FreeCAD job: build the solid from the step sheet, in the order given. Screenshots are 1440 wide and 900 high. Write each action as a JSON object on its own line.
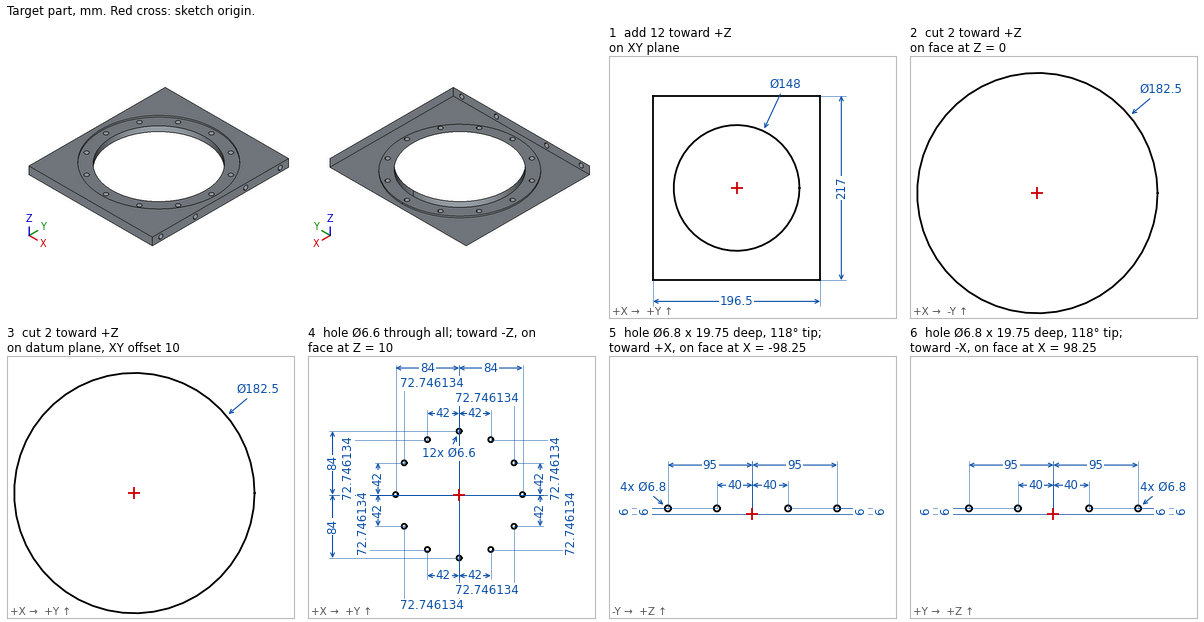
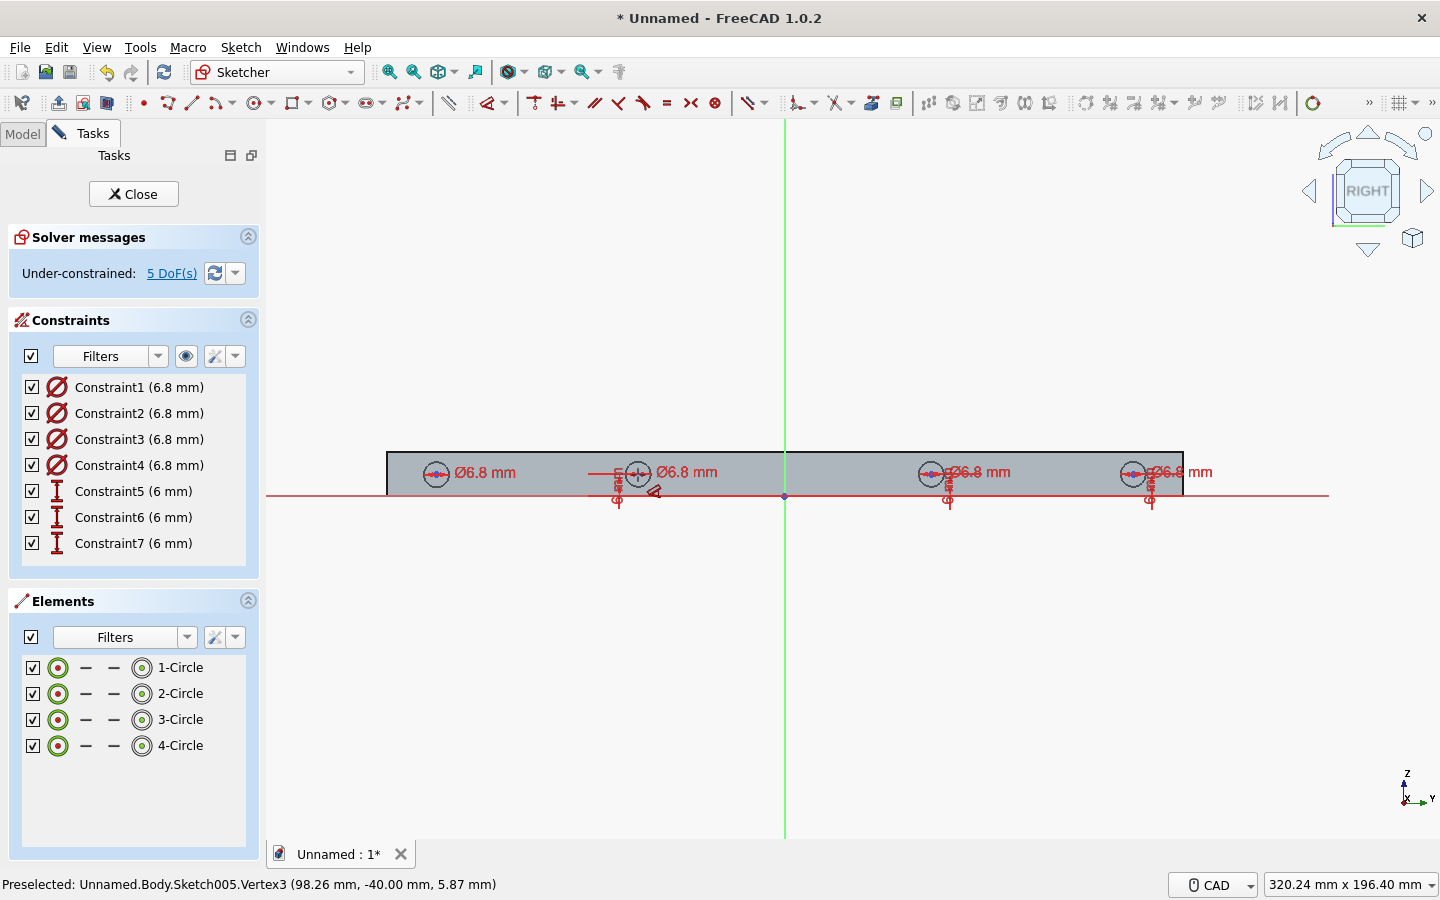
{"action": "scroll", "coordinate": [437, 475], "scroll_direction": "up", "scroll_amount": 3}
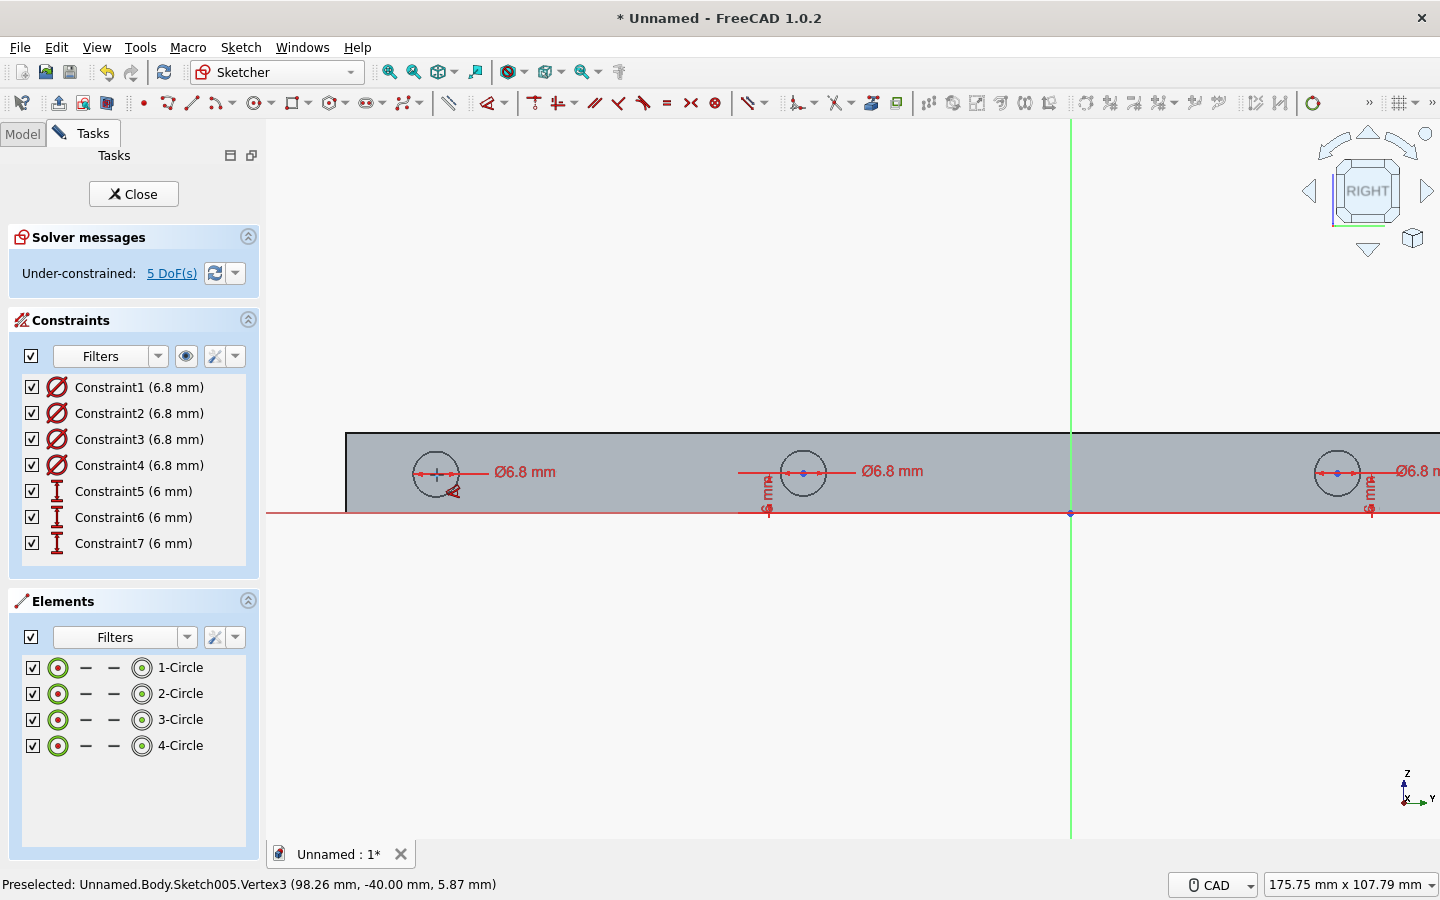
{"action": "left_click", "coordinate": [436, 474]}
{"action": "left_click", "coordinate": [402, 494]}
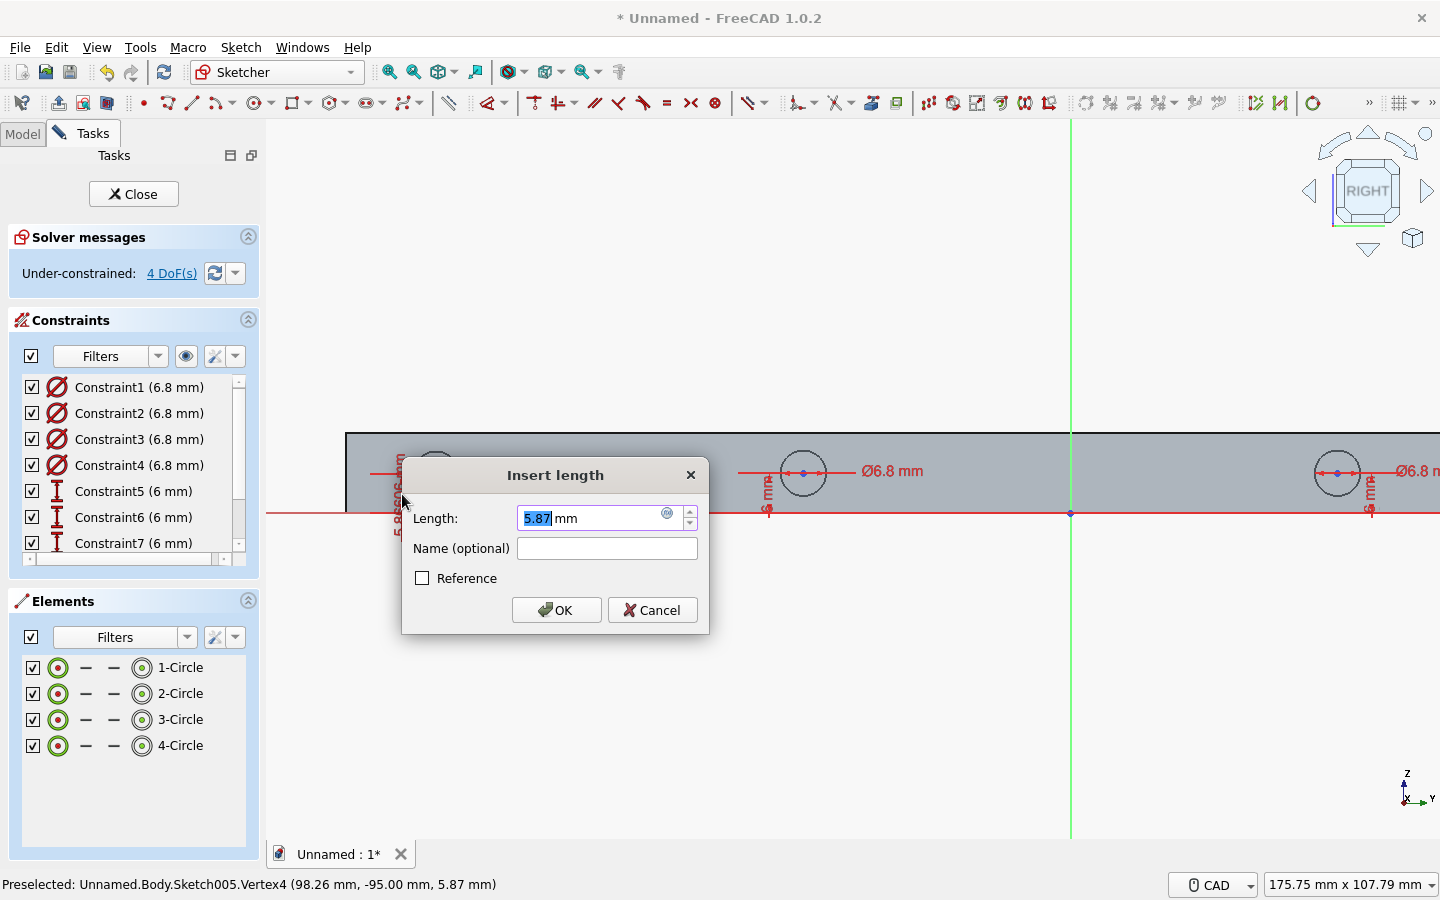
{"action": "type", "text": "6"}
{"action": "key", "text": "Return"}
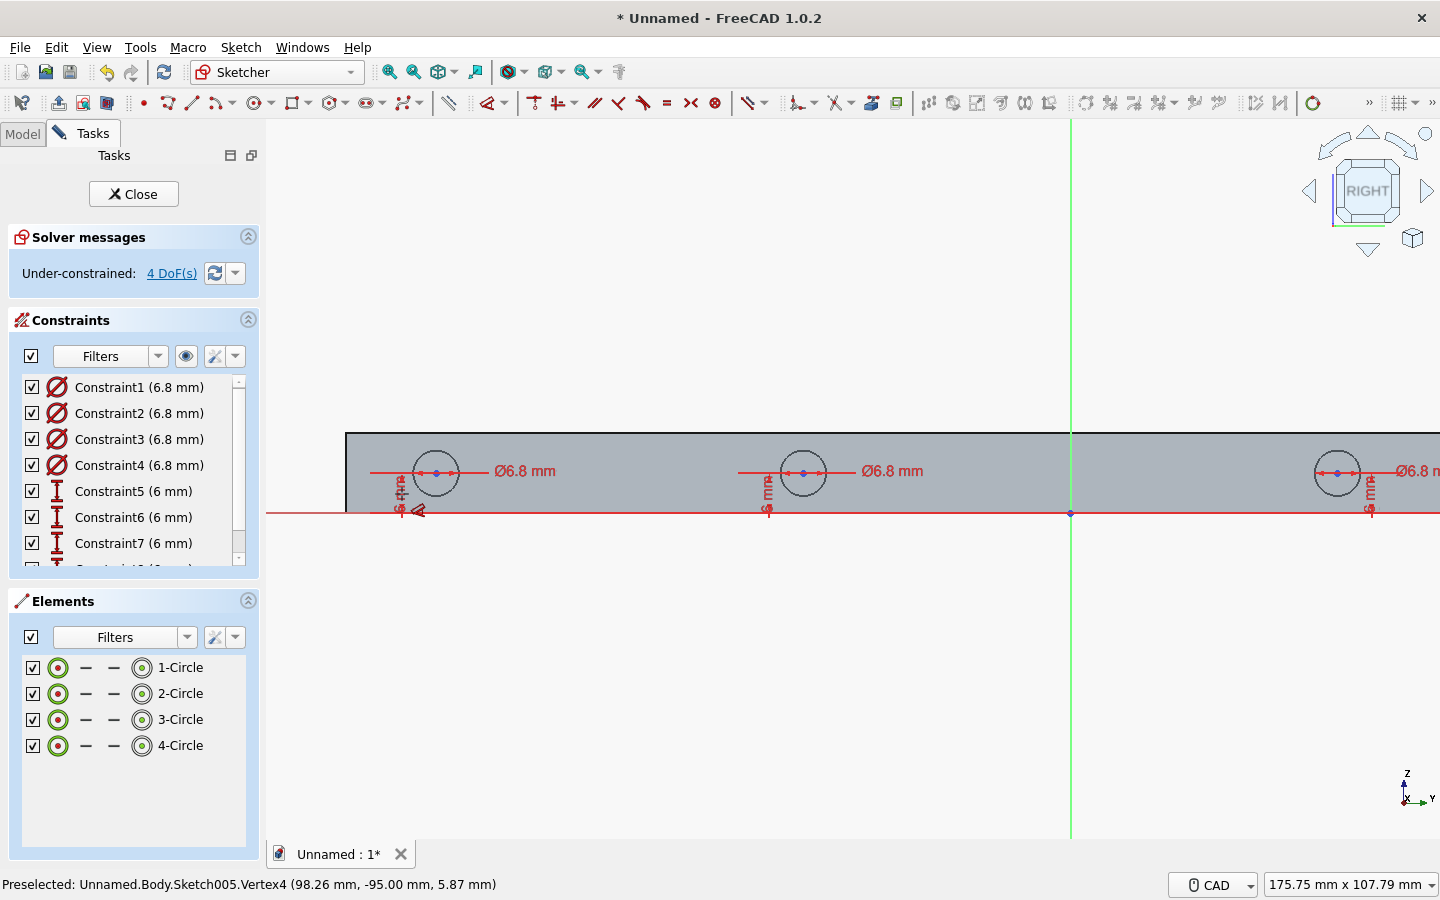
{"action": "scroll", "coordinate": [437, 475], "scroll_direction": "down", "scroll_amount": 3}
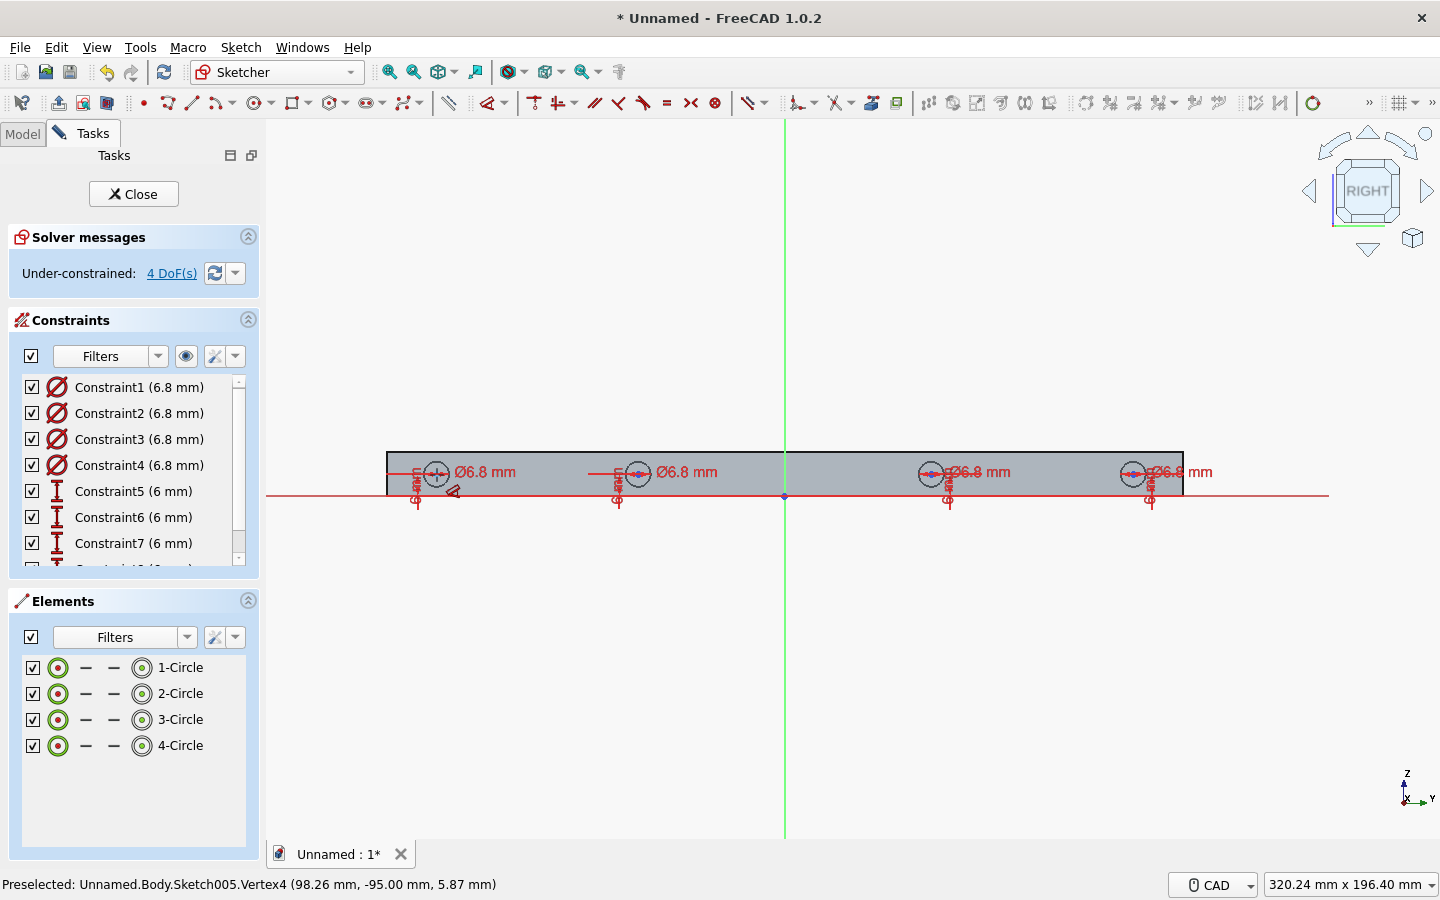
{"action": "left_click", "coordinate": [1133, 474]}
{"action": "left_click", "coordinate": [959, 530]}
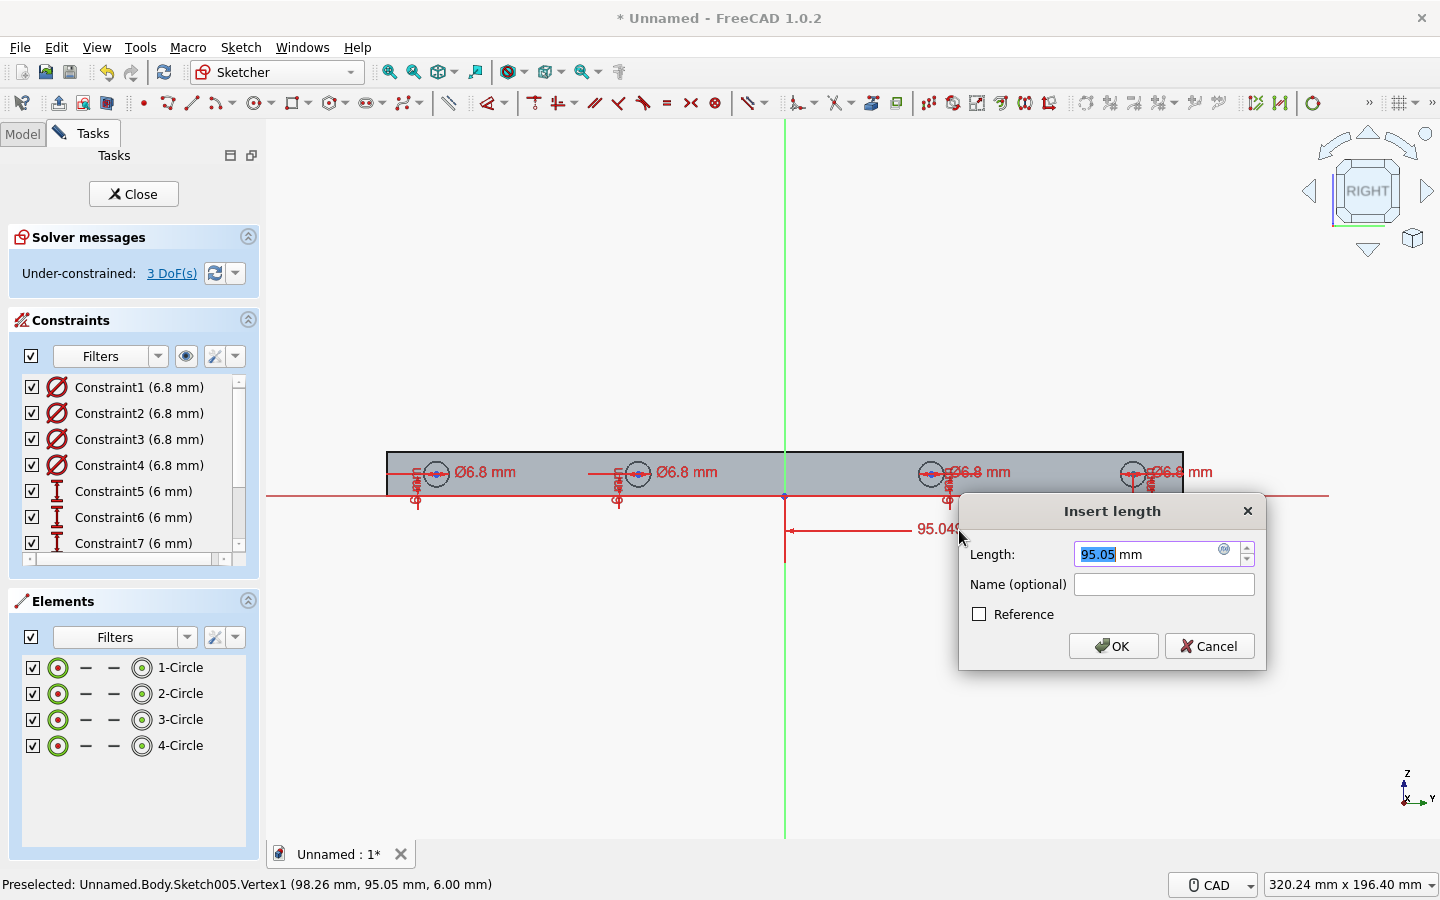
{"action": "type", "text": "95"}
{"action": "key", "text": "Return"}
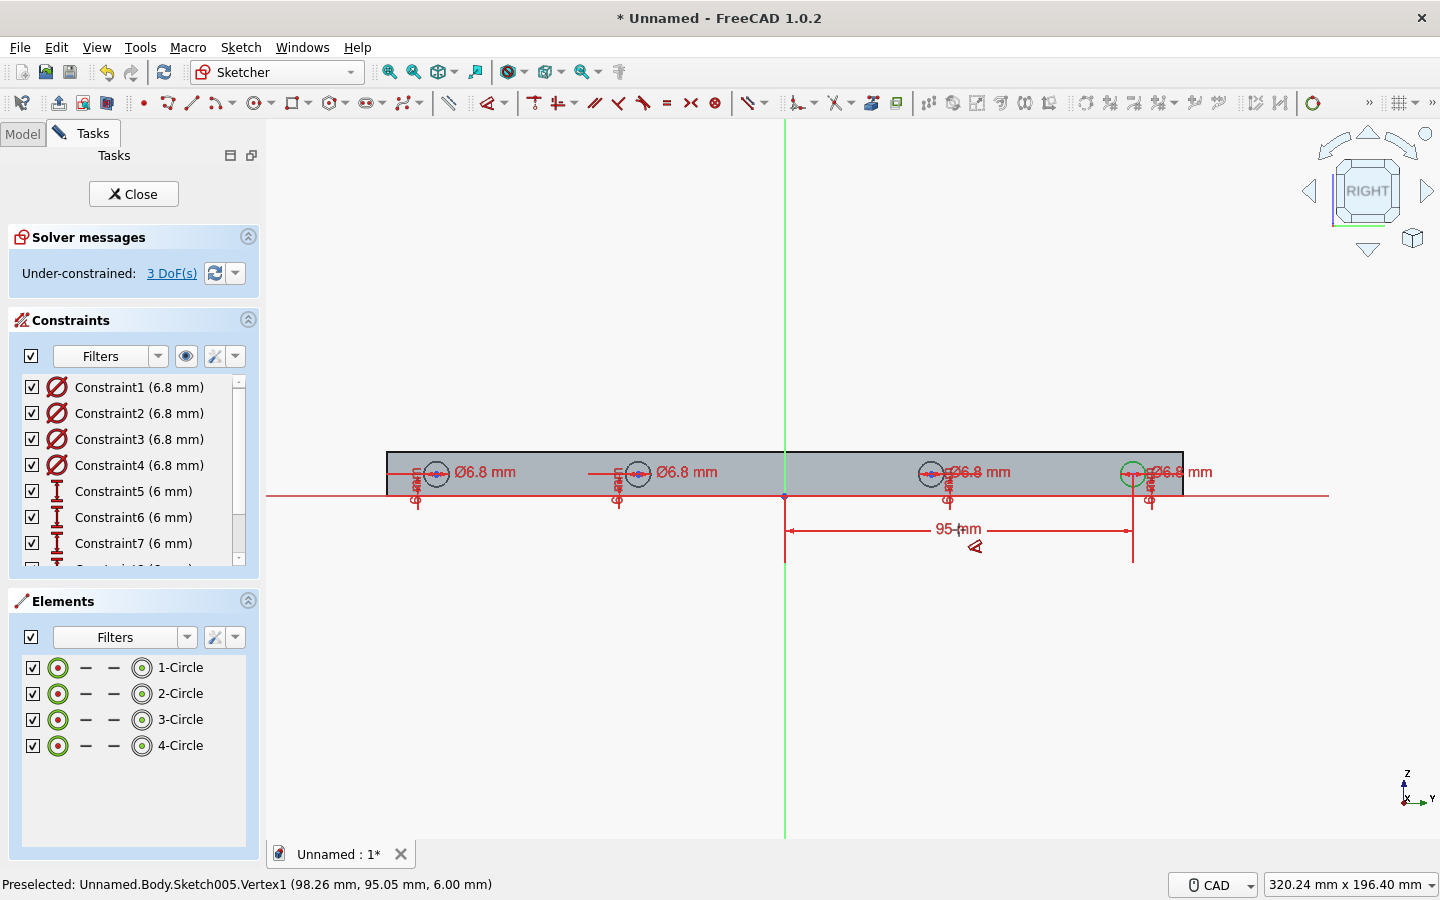
{"action": "left_click", "coordinate": [931, 474]}
{"action": "left_click", "coordinate": [858, 530]}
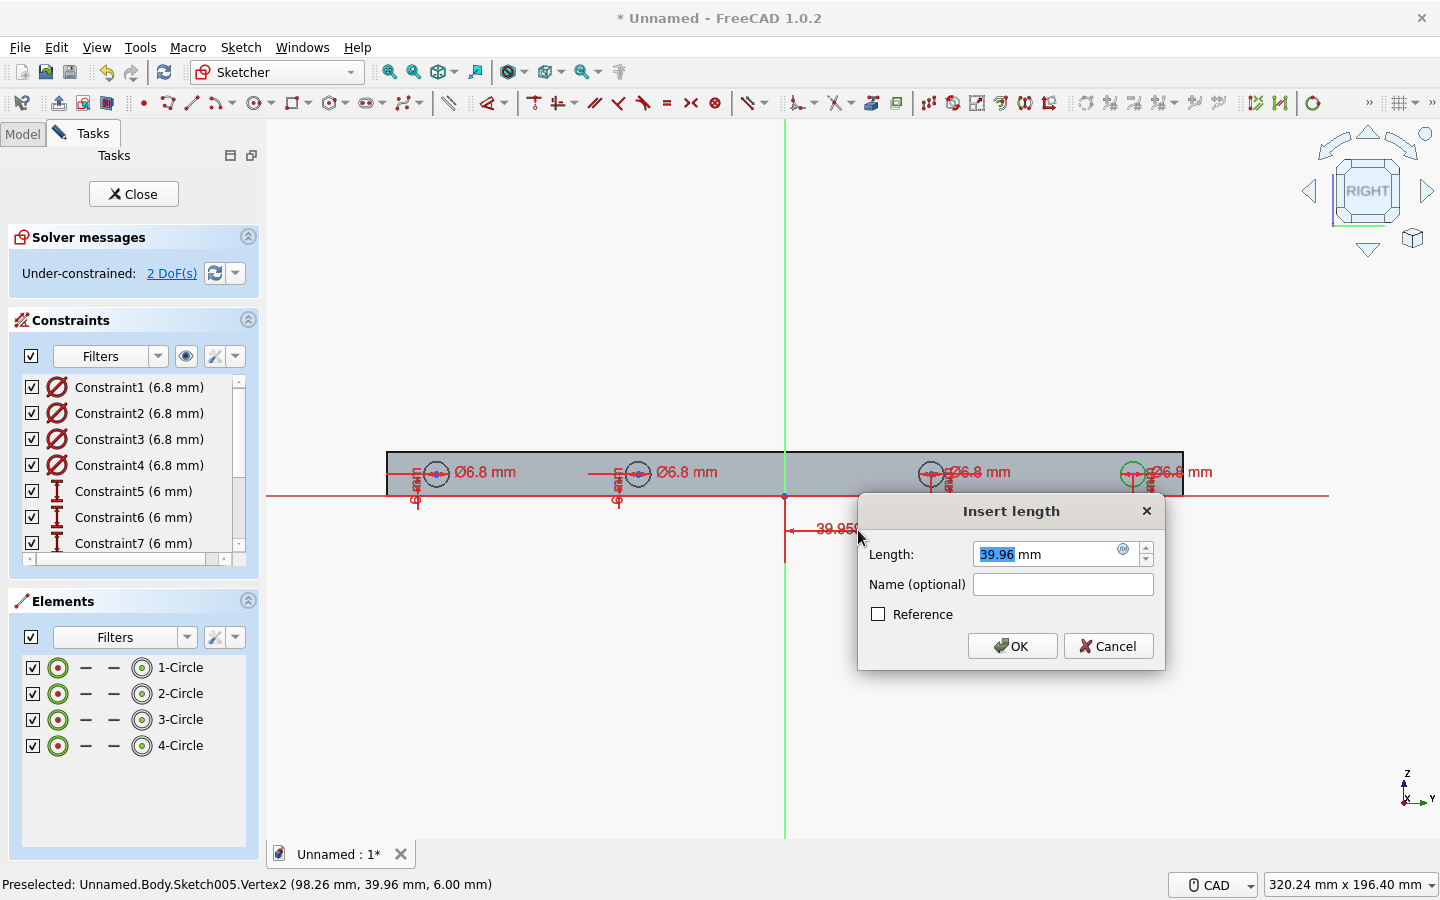
{"action": "type", "text": "40"}
{"action": "key", "text": "Return"}